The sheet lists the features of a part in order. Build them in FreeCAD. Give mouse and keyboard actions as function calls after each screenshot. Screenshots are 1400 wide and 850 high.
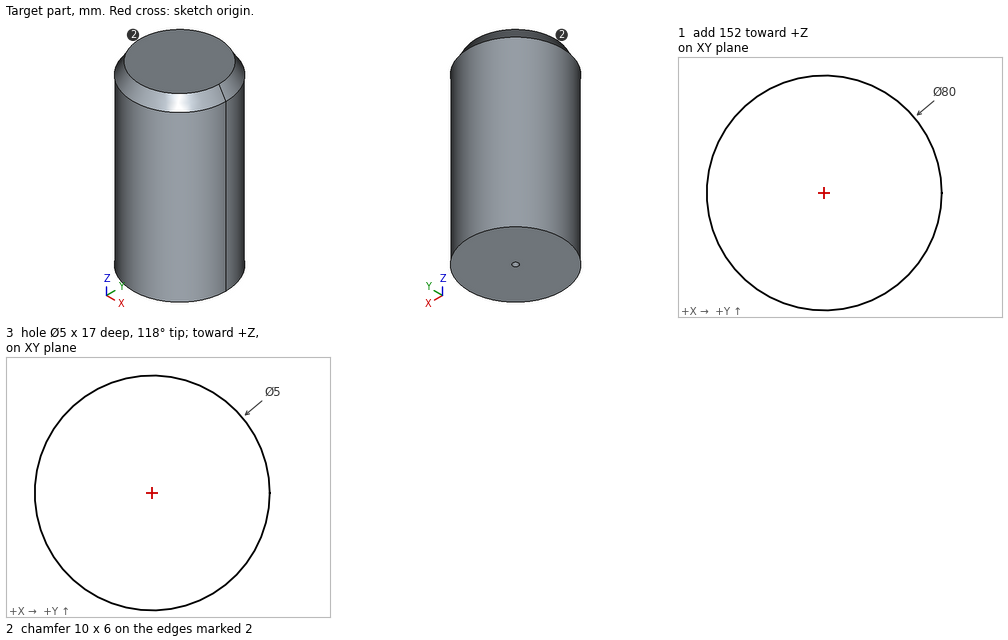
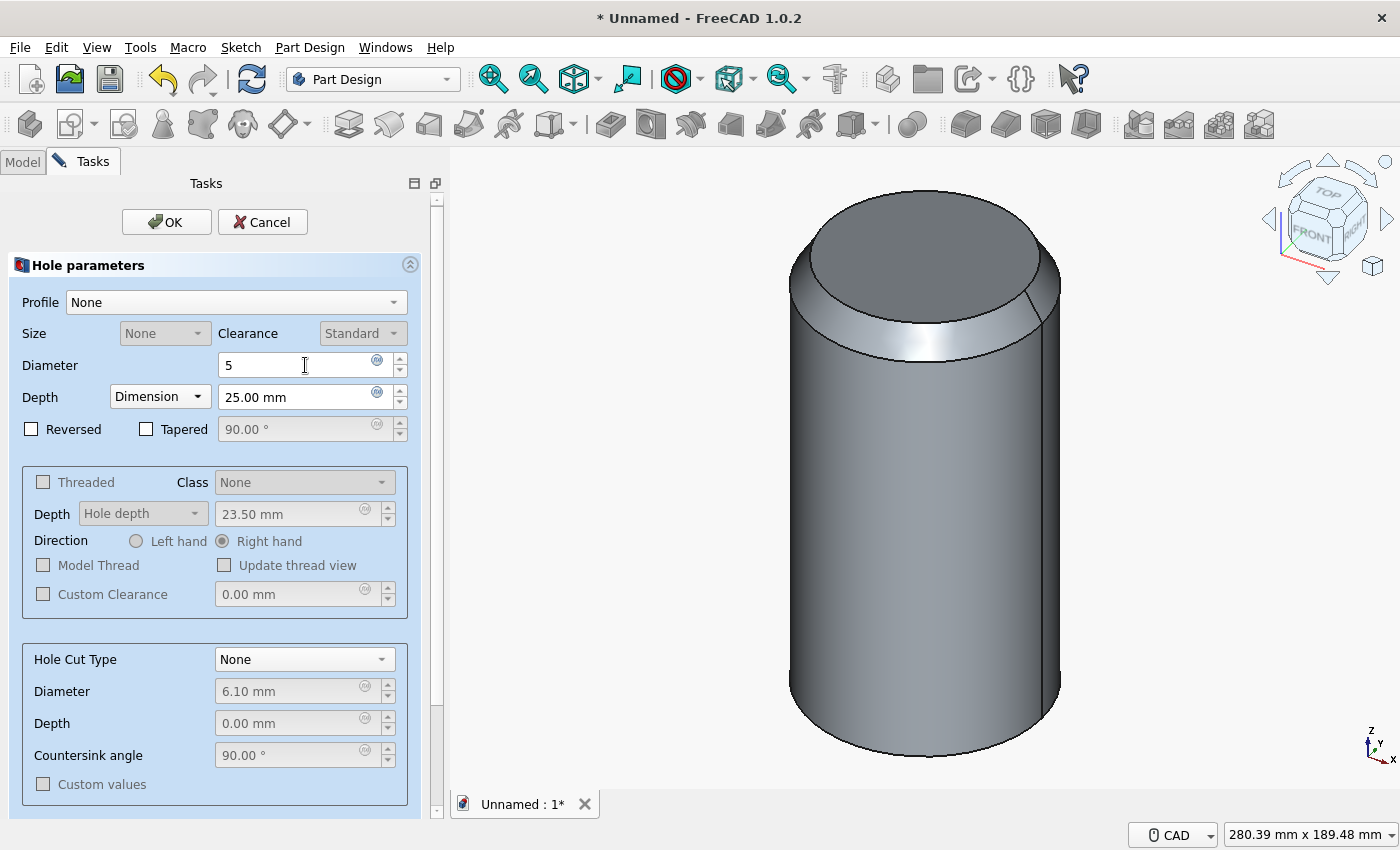
triple_click(305, 397)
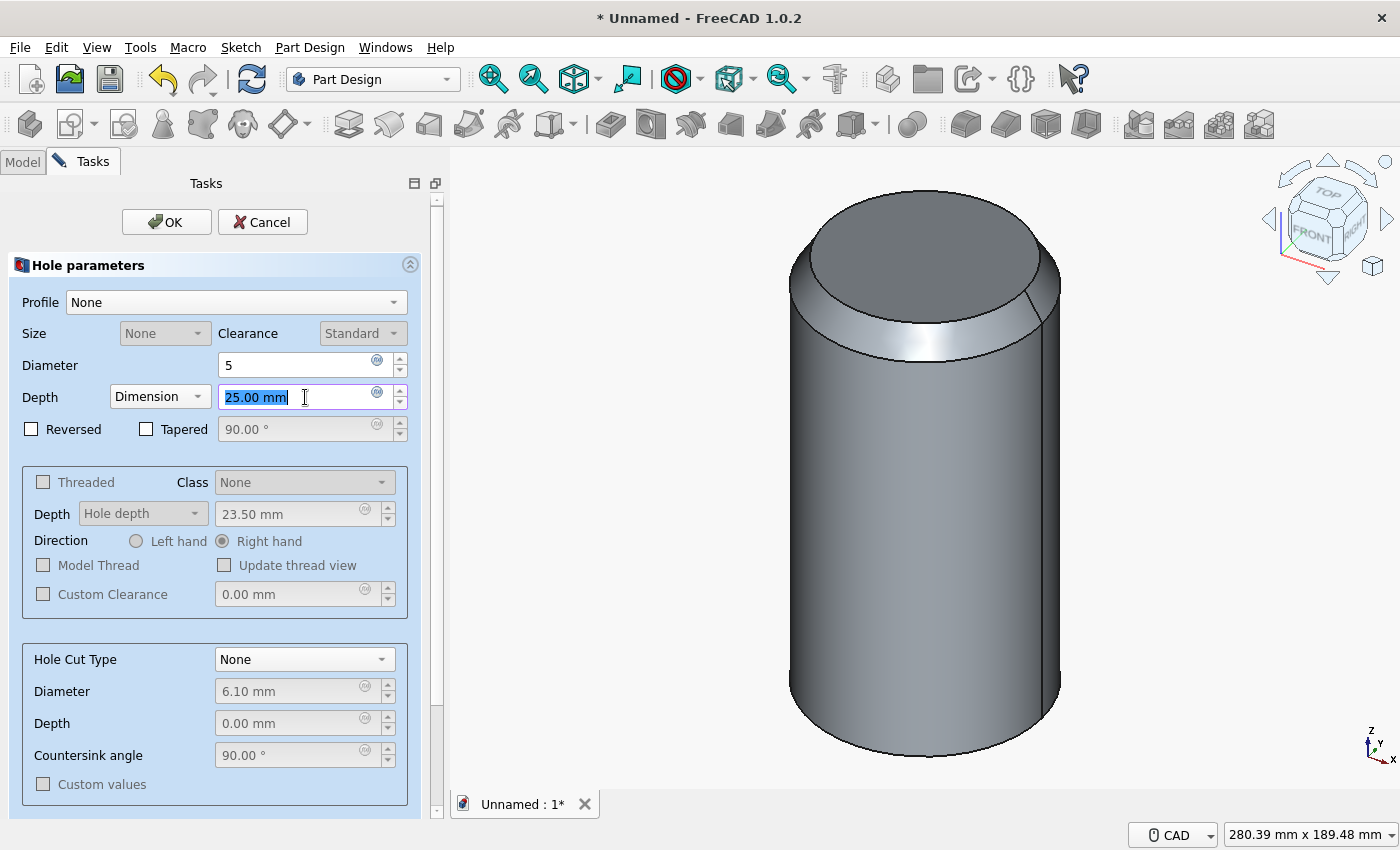
text(17)
key(Tab)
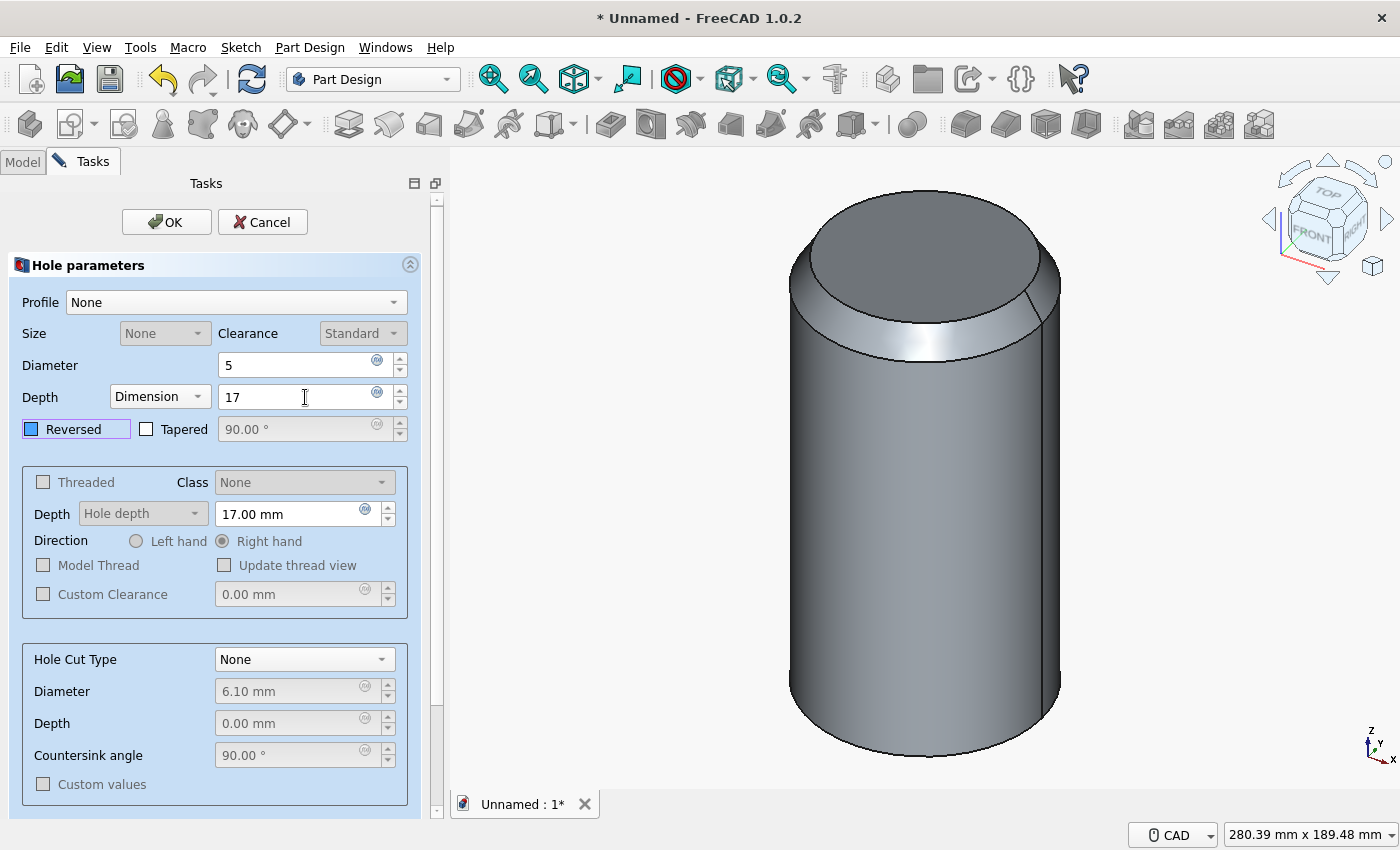
click(30, 429)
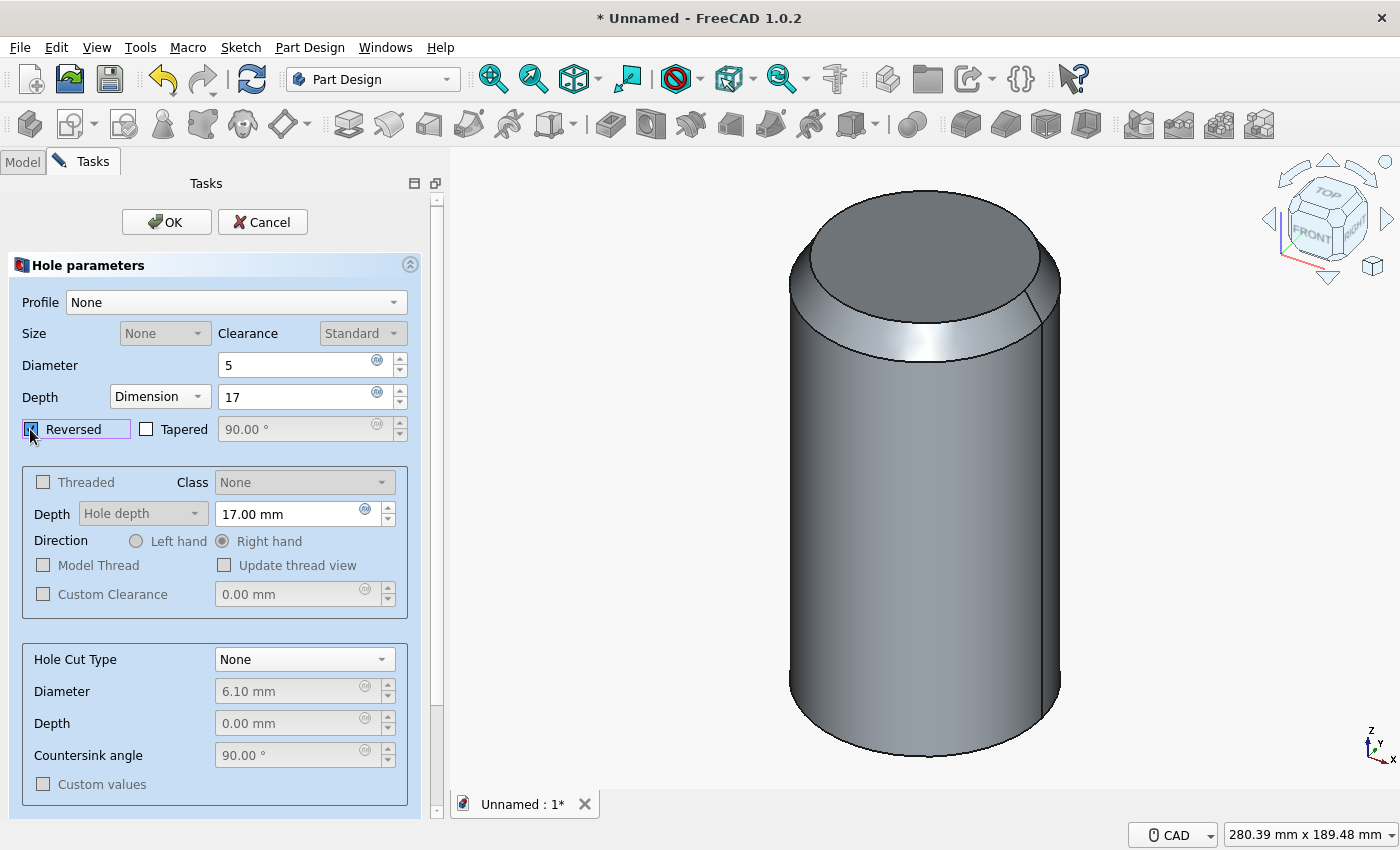
click(167, 222)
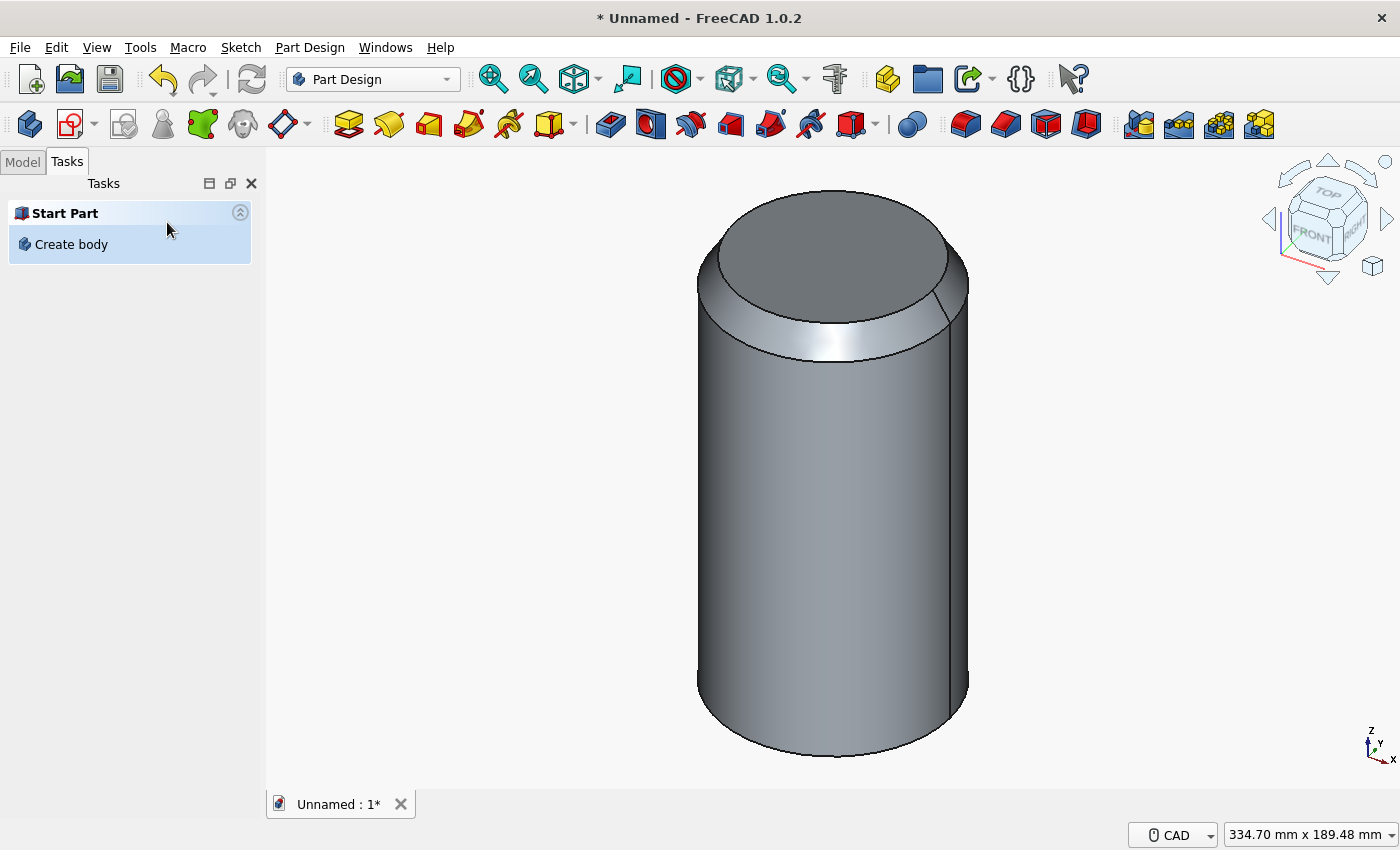
key(0)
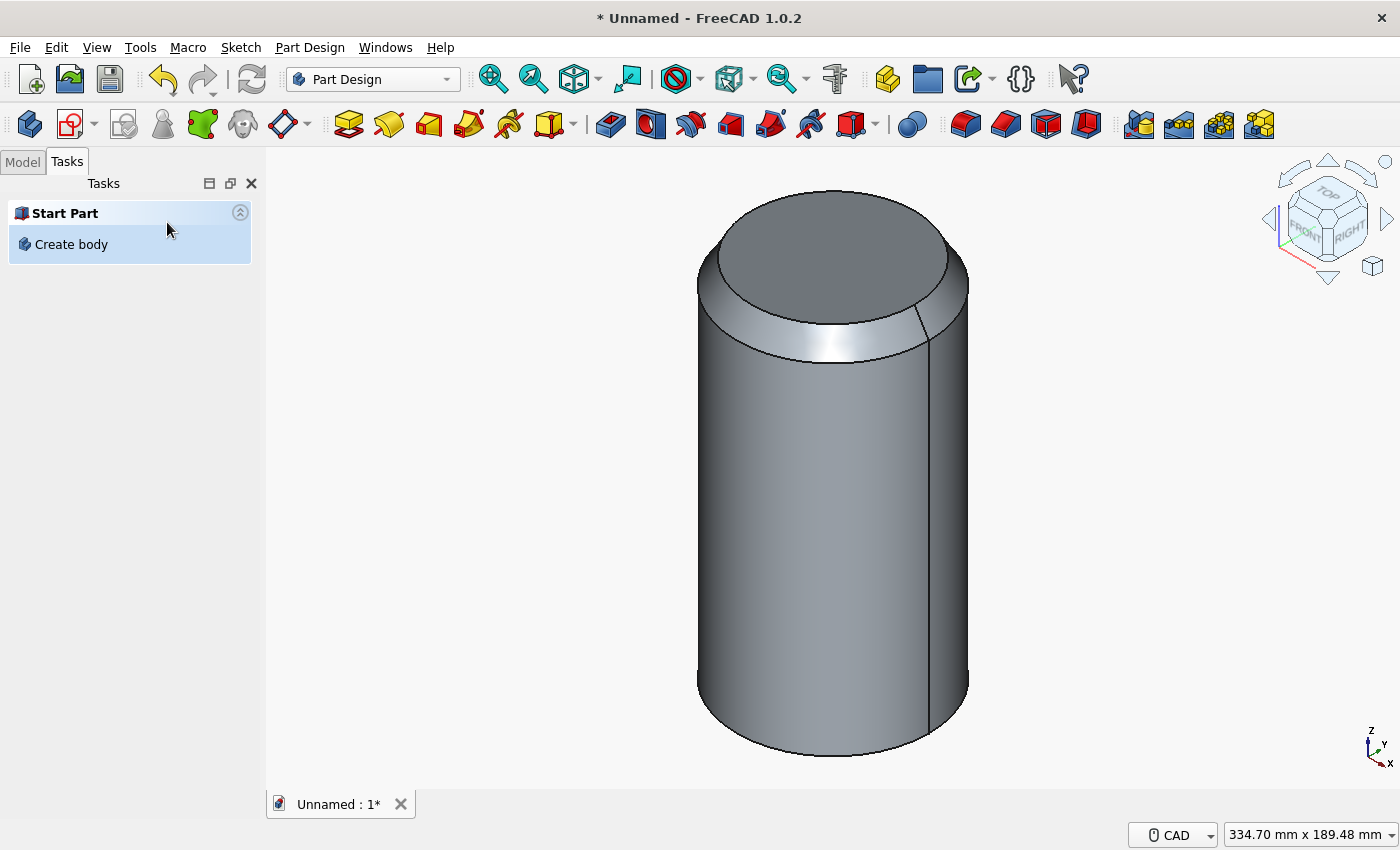
click(494, 80)